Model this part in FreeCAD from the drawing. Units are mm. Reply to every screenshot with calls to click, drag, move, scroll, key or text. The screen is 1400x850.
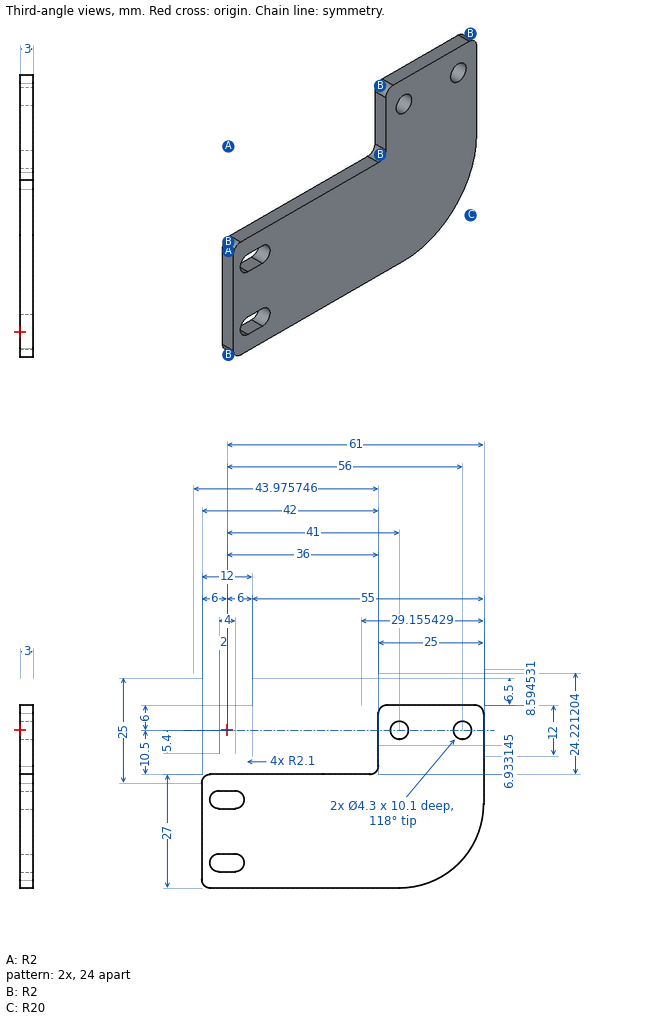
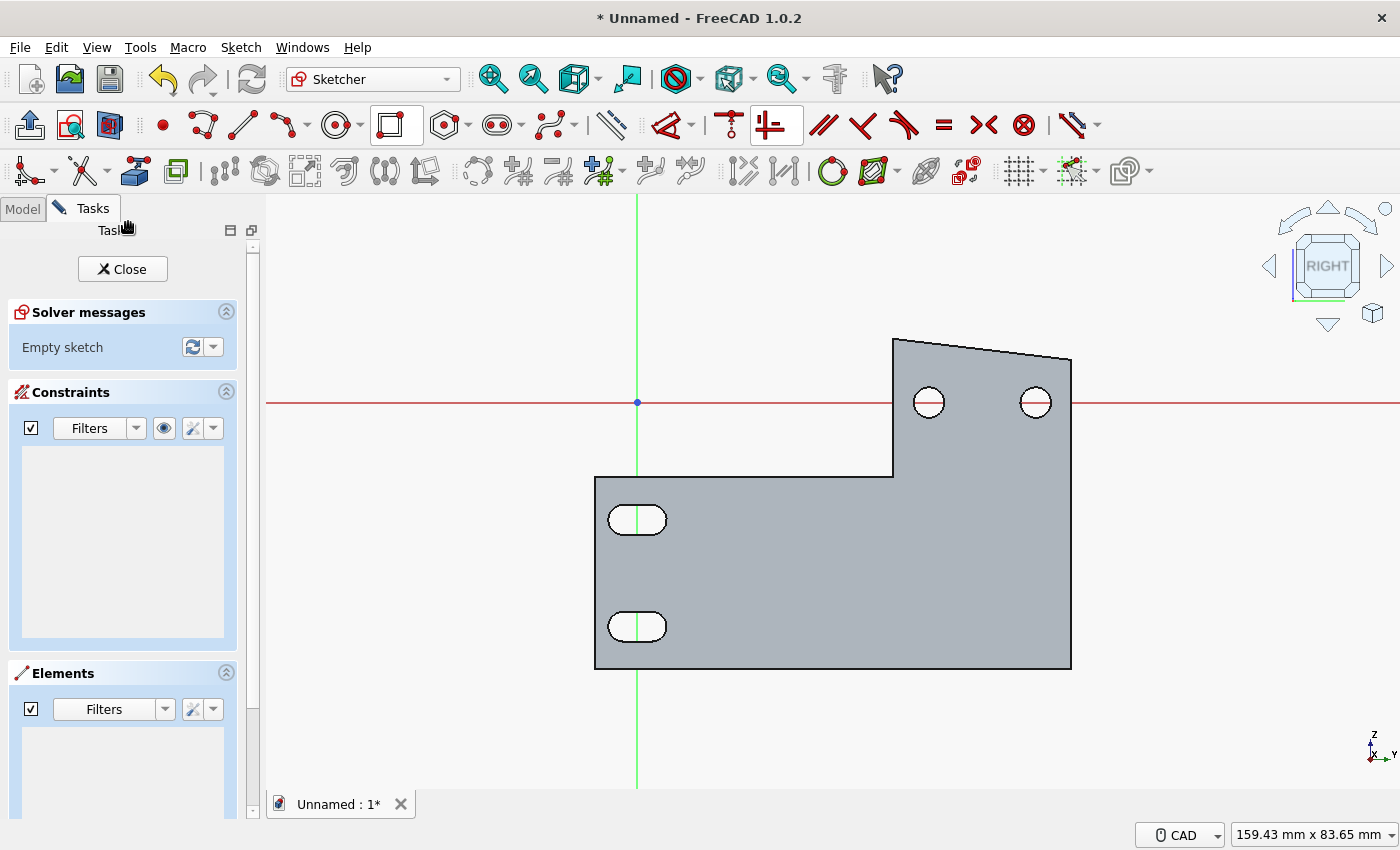
click(110, 126)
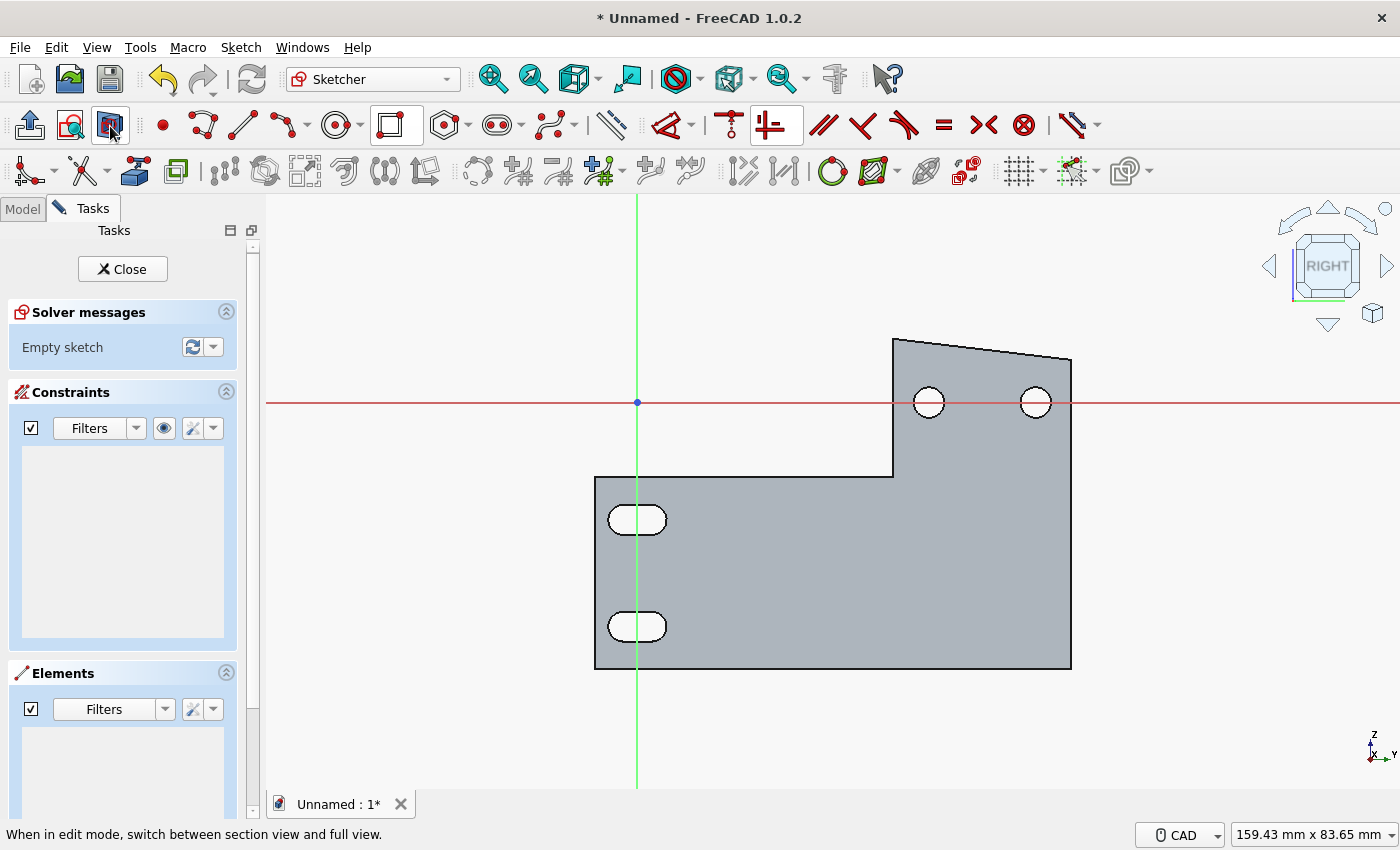
scroll(1037, 222, up, 2)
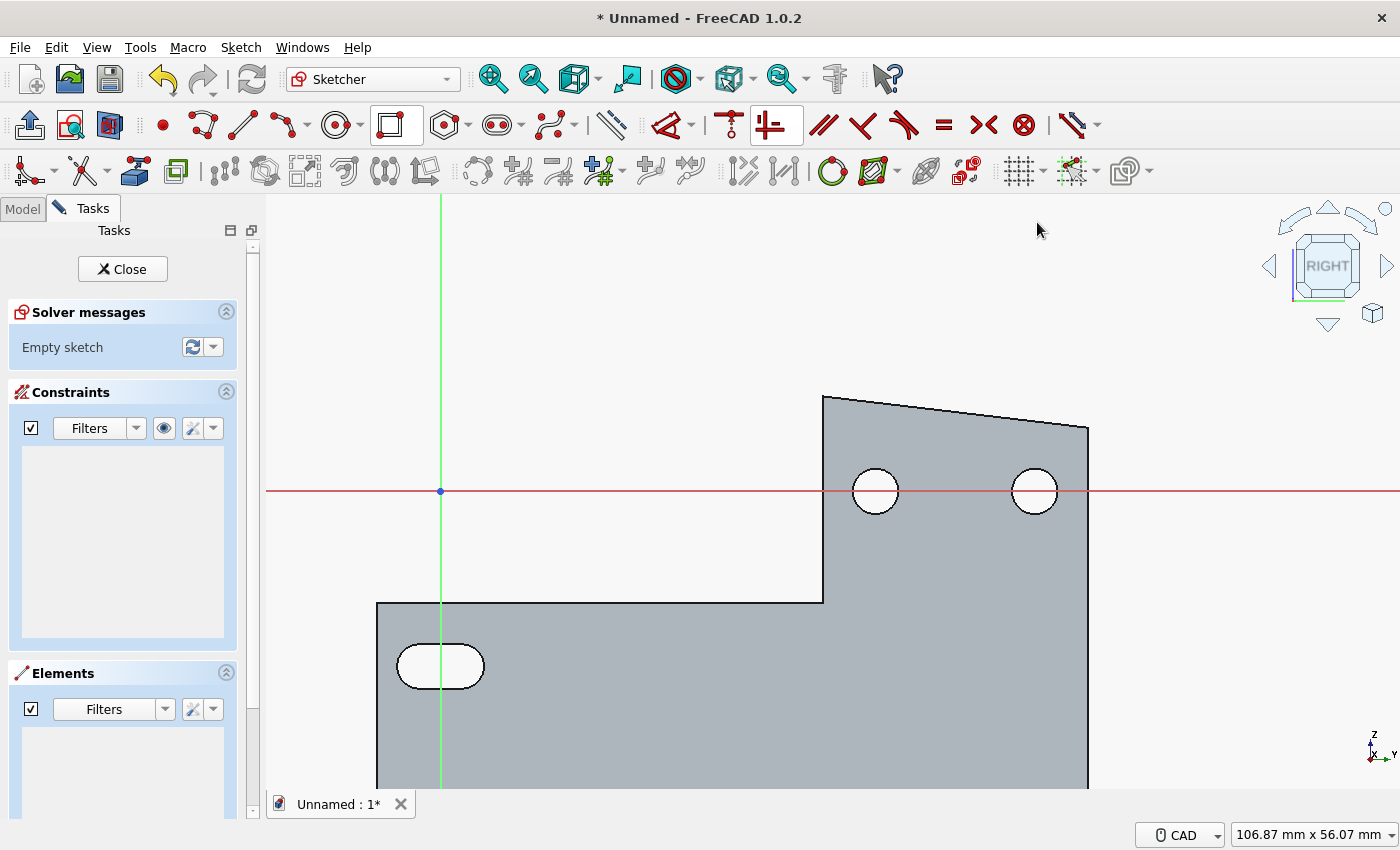
click(390, 126)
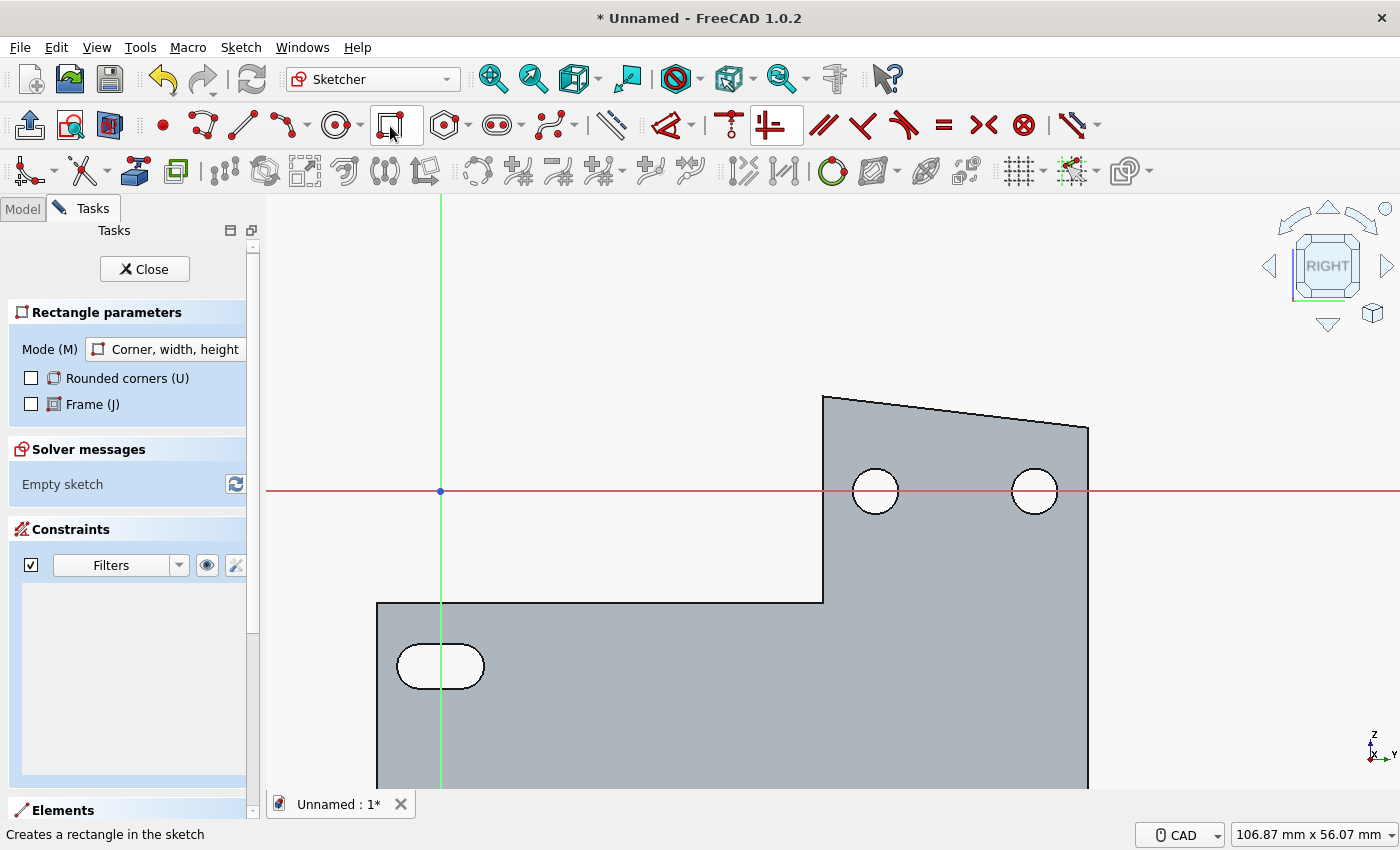
click(778, 337)
move(1088, 428)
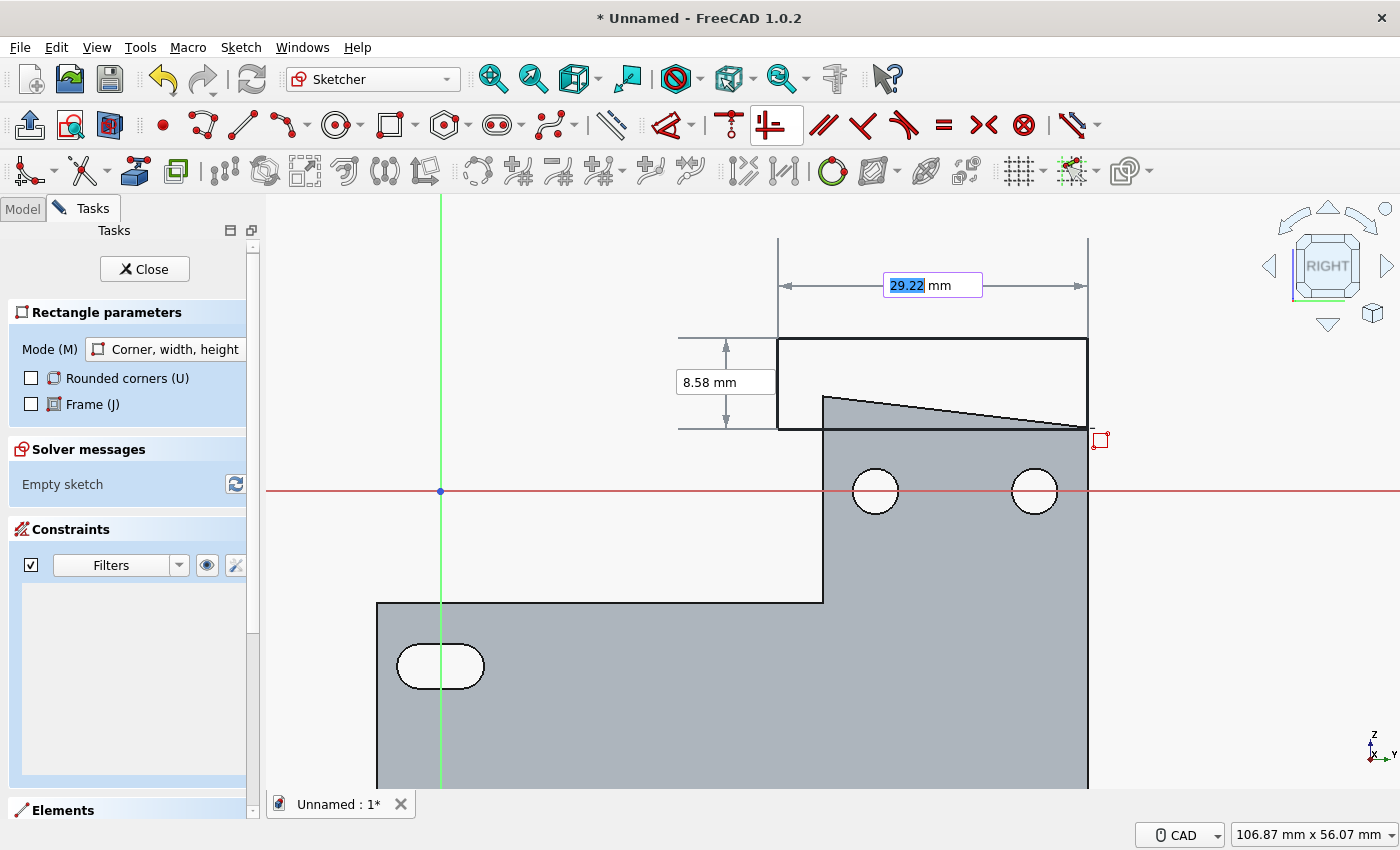
text(29.155429)
key(Tab)
text(8.594531)
key(Return)
key(Escape)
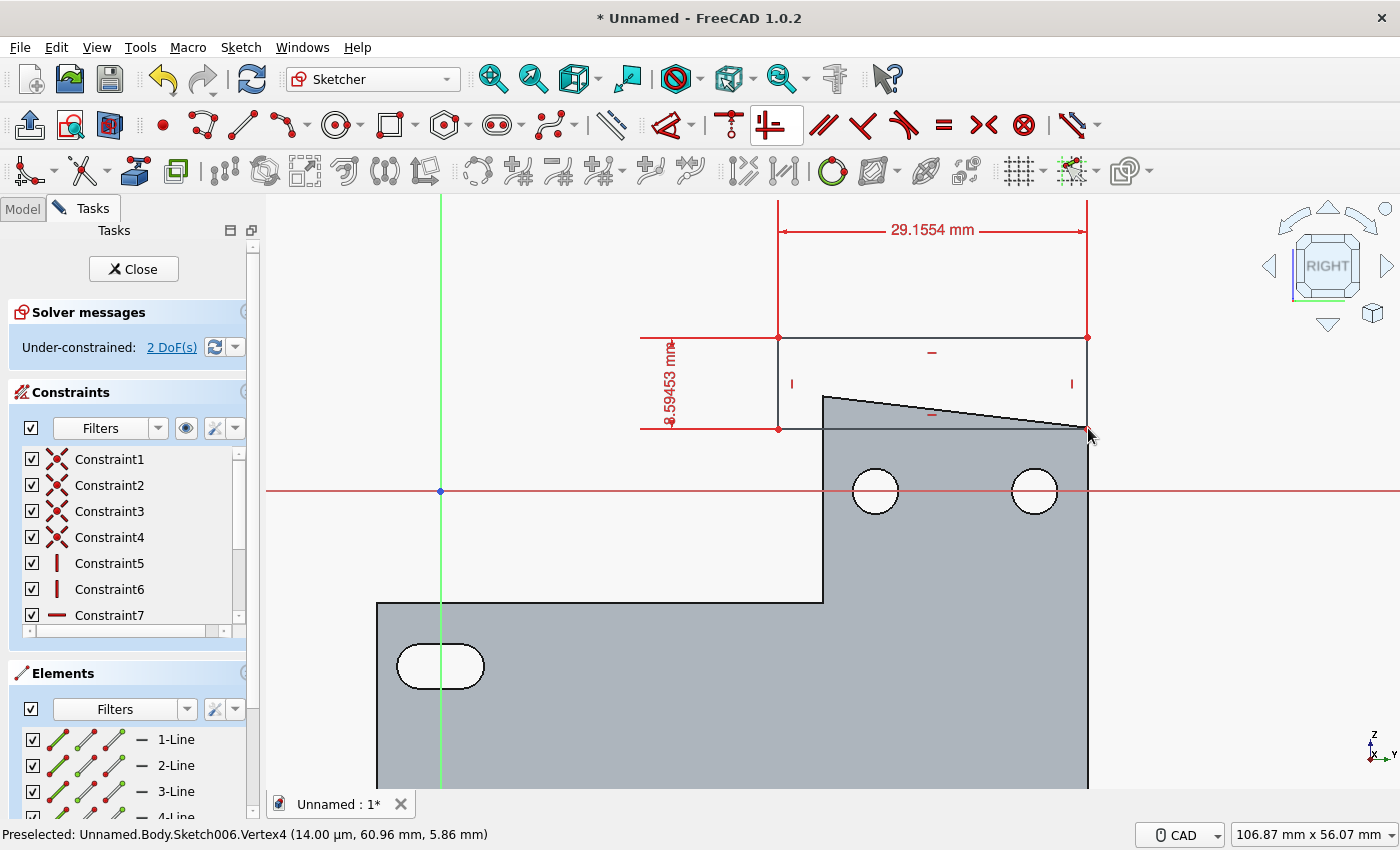
click(666, 126)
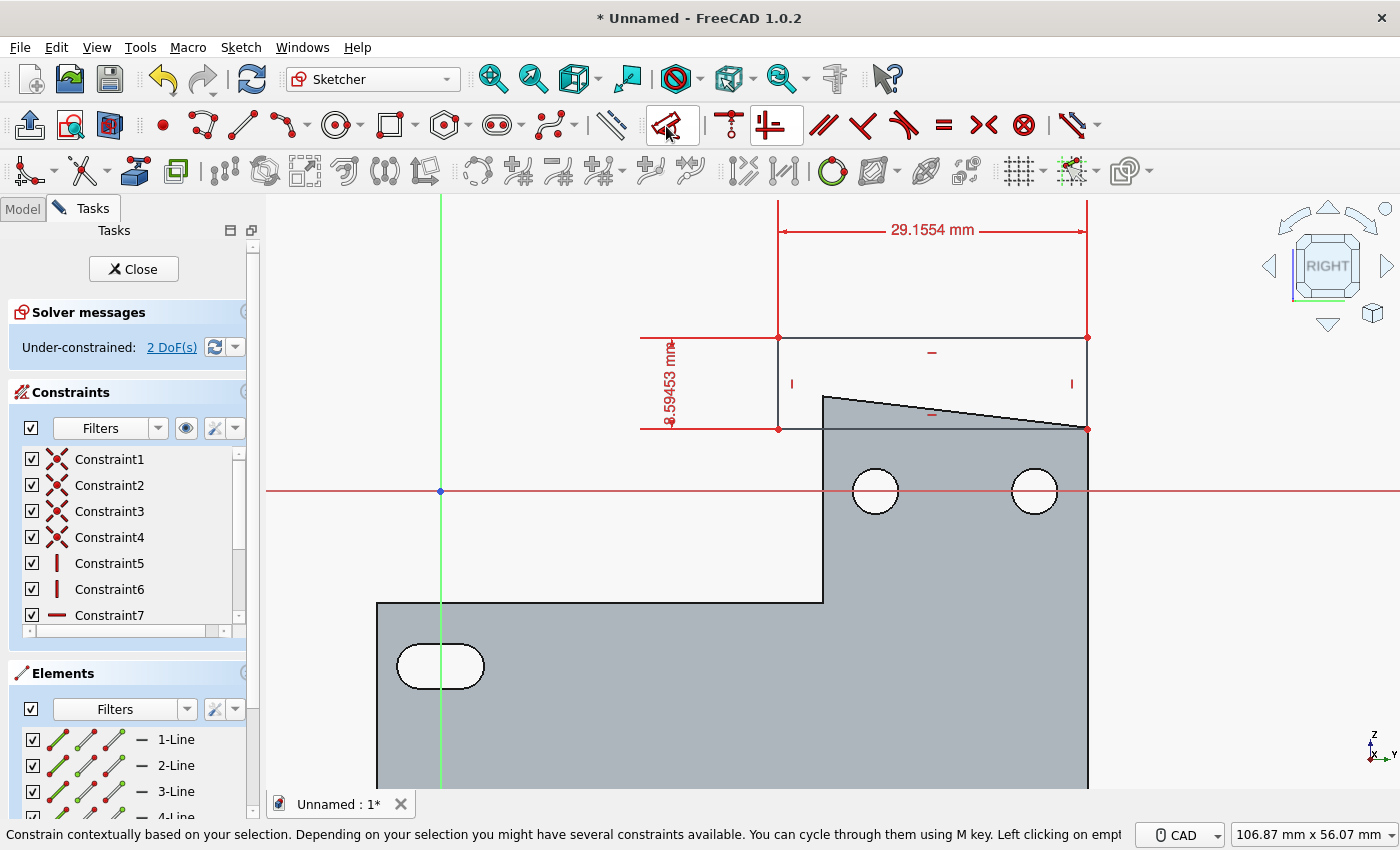
click(778, 429)
click(407, 460)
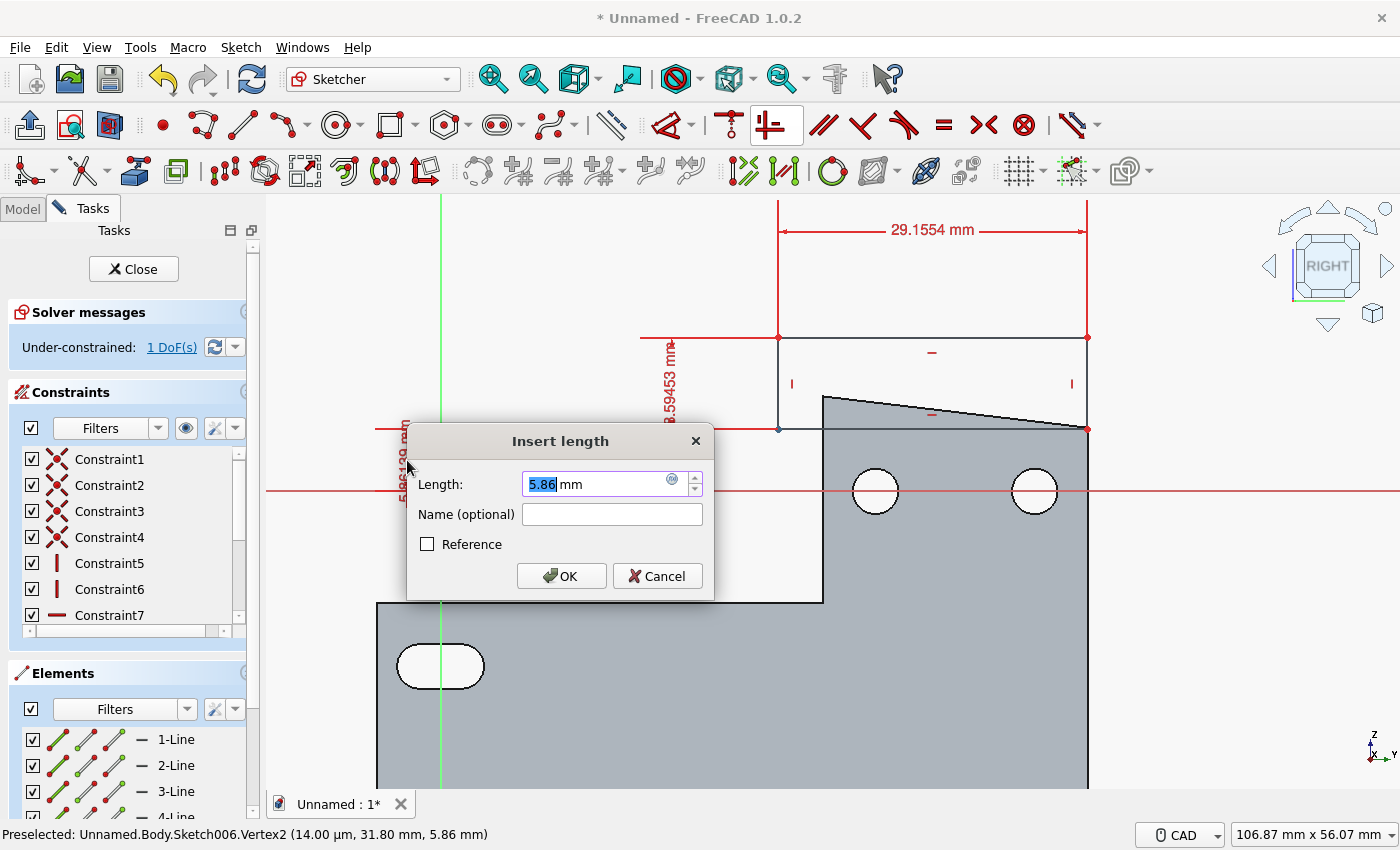
text(6)
key(Return)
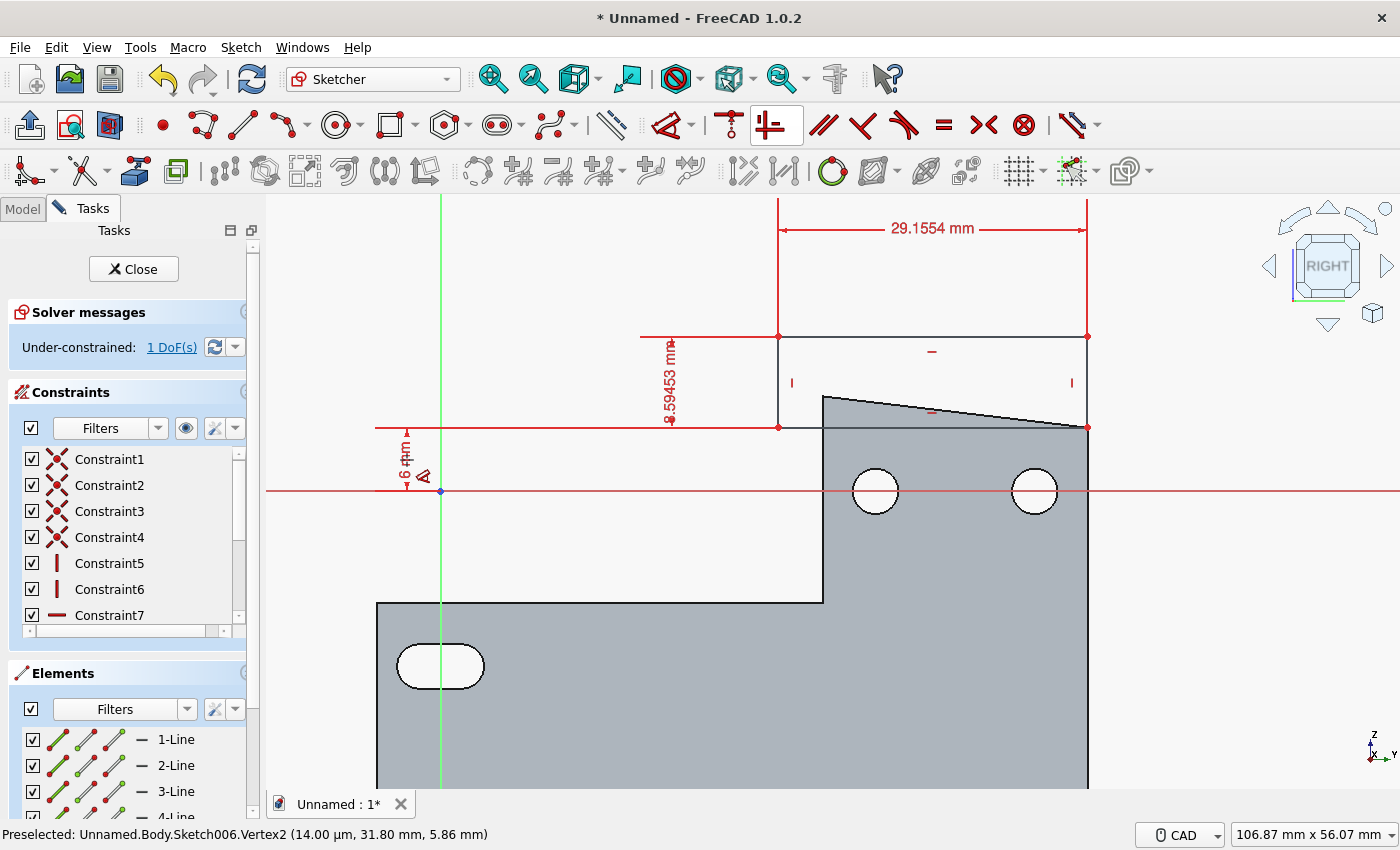
click(1087, 428)
click(764, 525)